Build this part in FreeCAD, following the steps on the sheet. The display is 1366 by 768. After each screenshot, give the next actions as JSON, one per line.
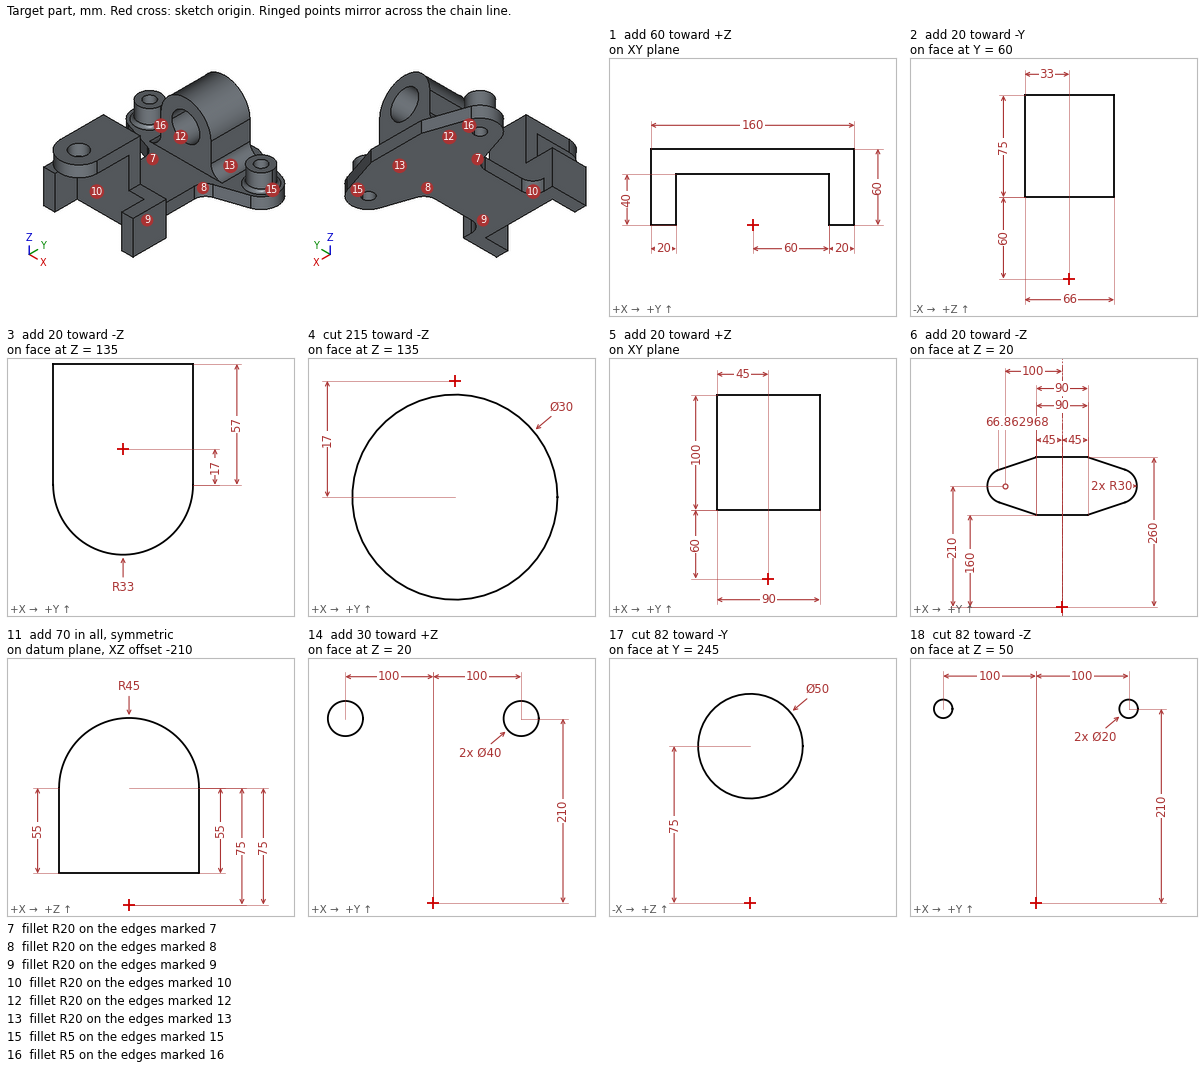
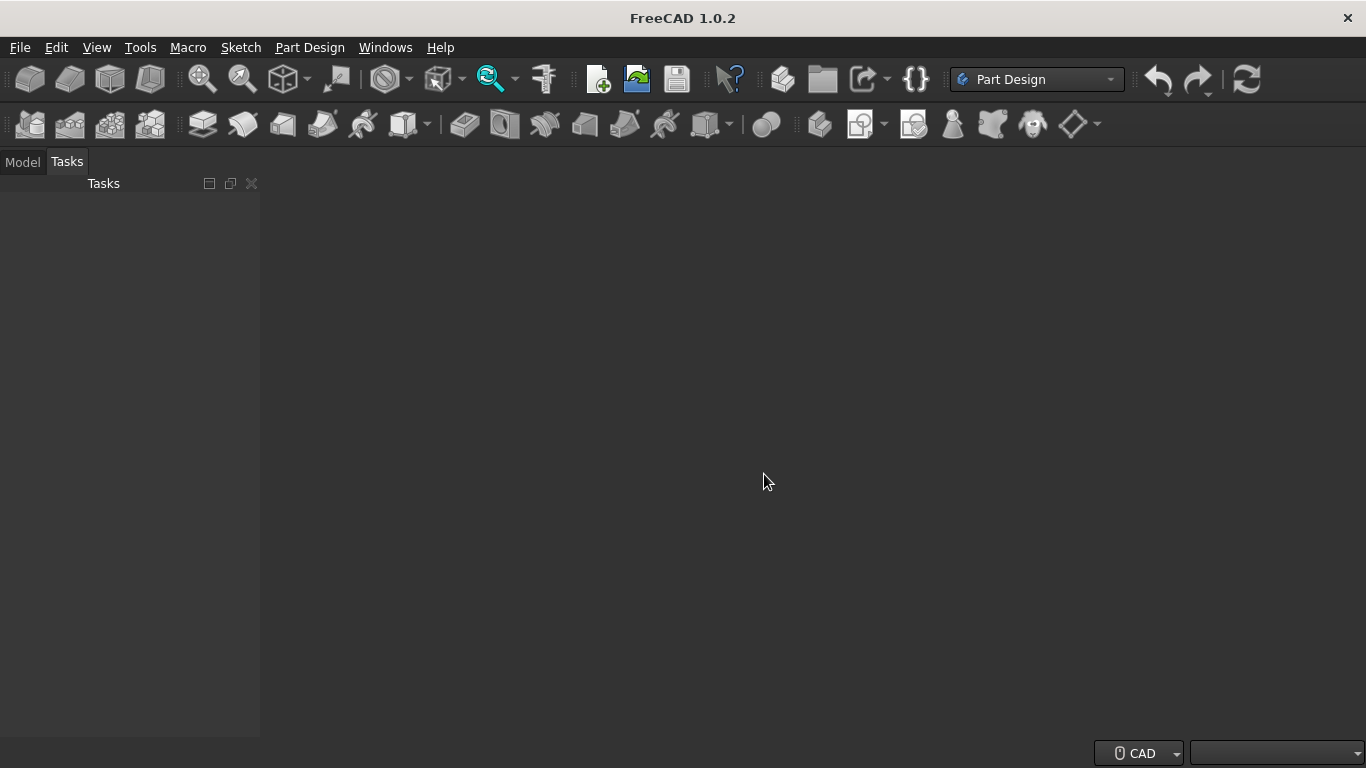
{"action": "key", "text": "ctrl+n"}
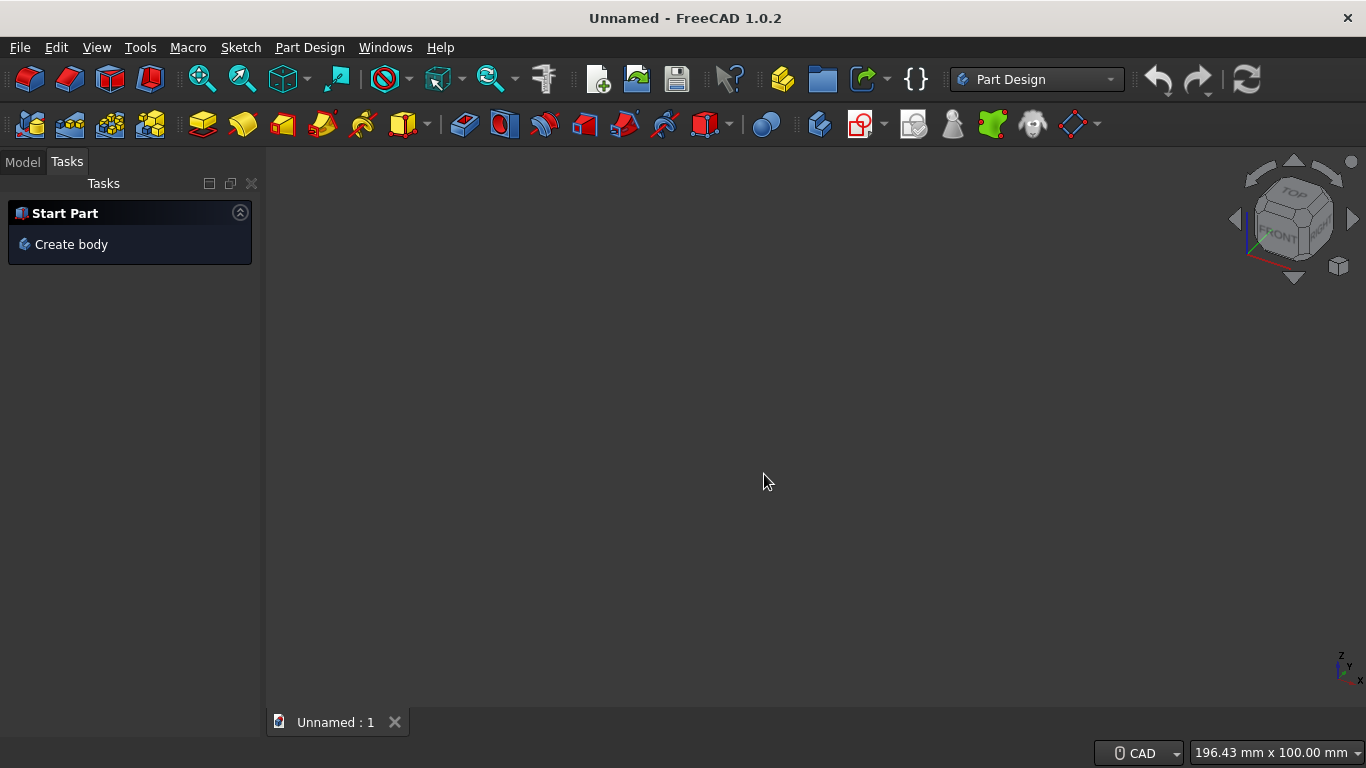
{"action": "left_click", "coordinate": [860, 124]}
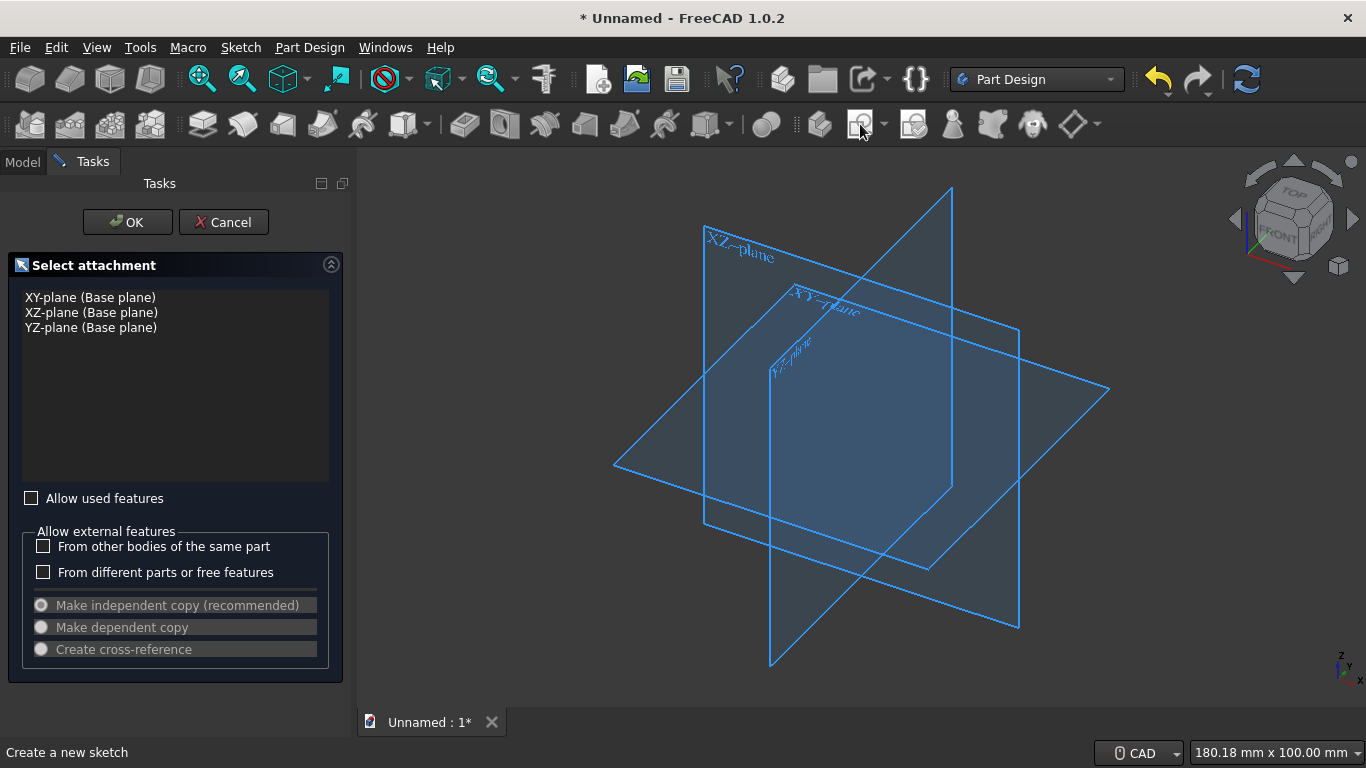
{"action": "left_click", "coordinate": [82, 298]}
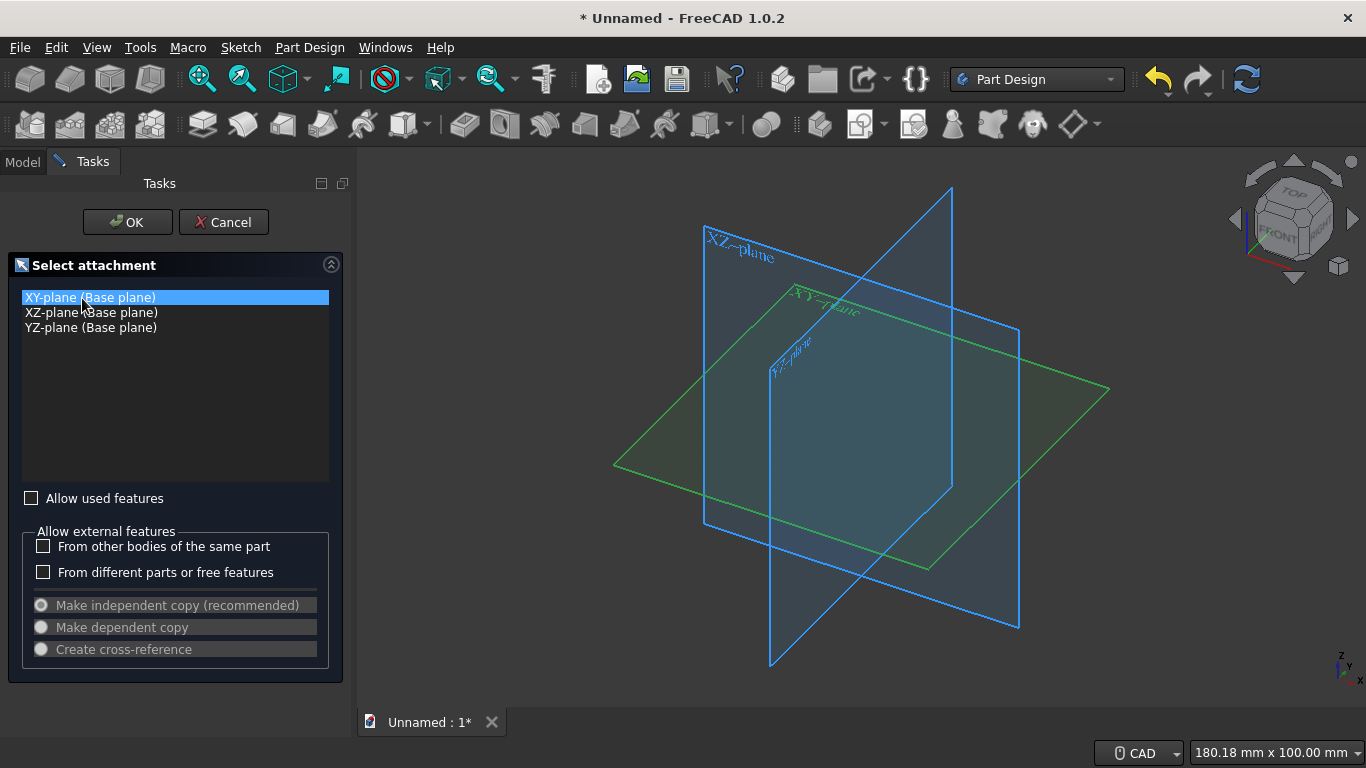
{"action": "left_click", "coordinate": [128, 222]}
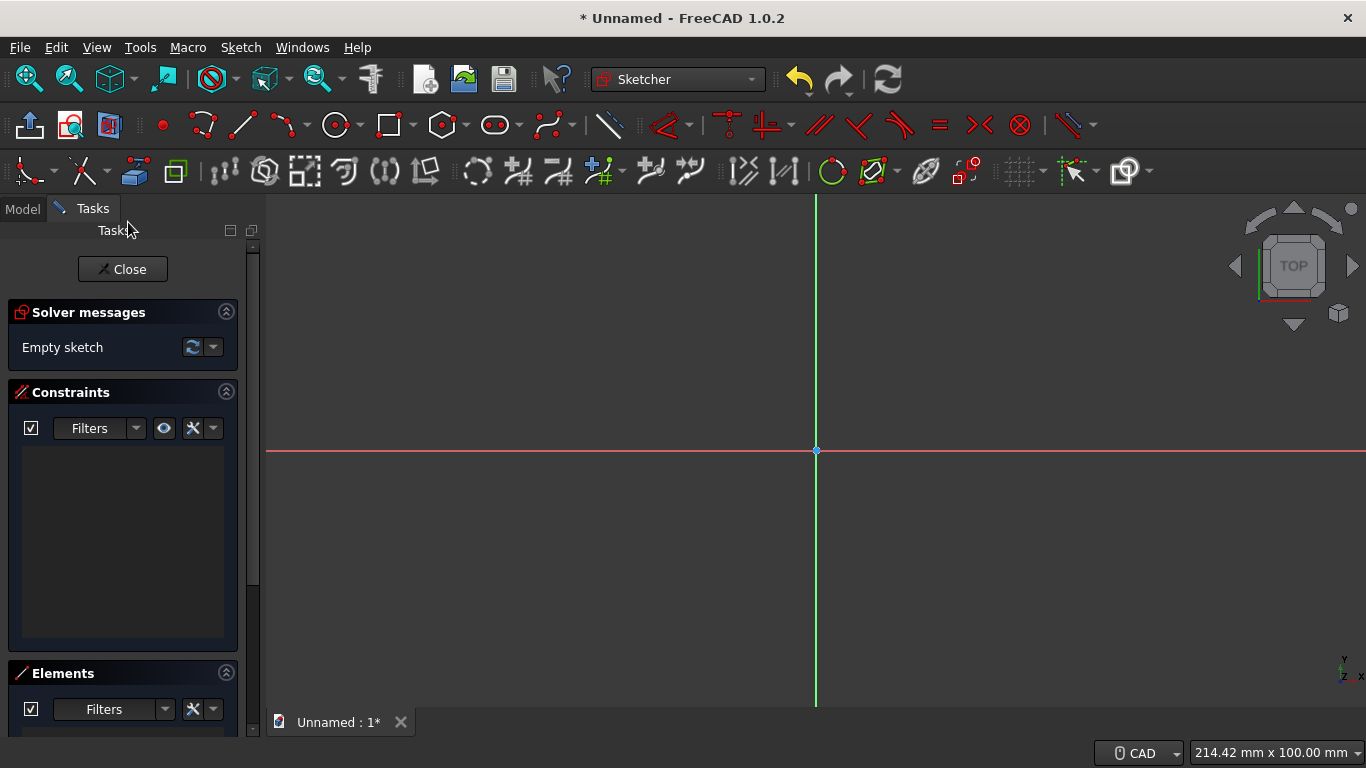
{"action": "scroll", "coordinate": [608, 679], "scroll_direction": "down", "scroll_amount": 2}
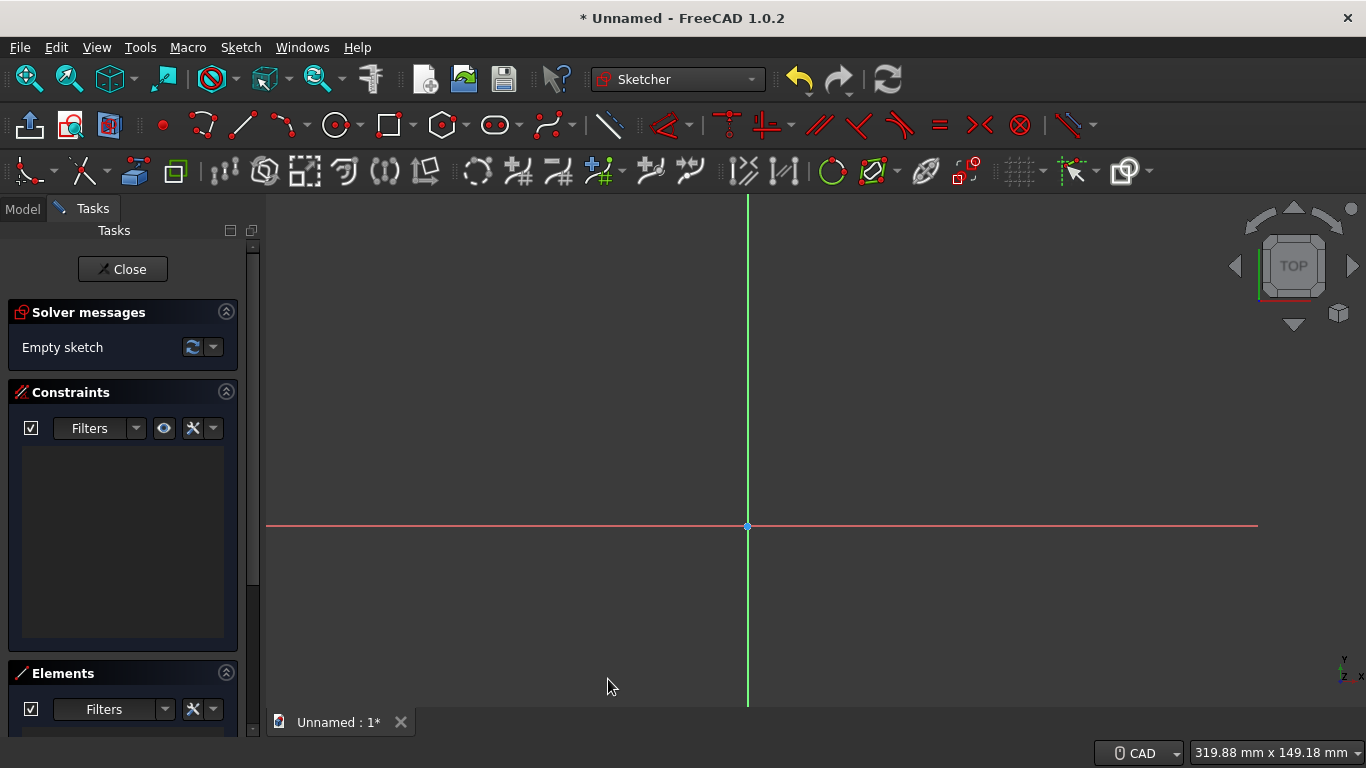
{"action": "key", "text": "g m"}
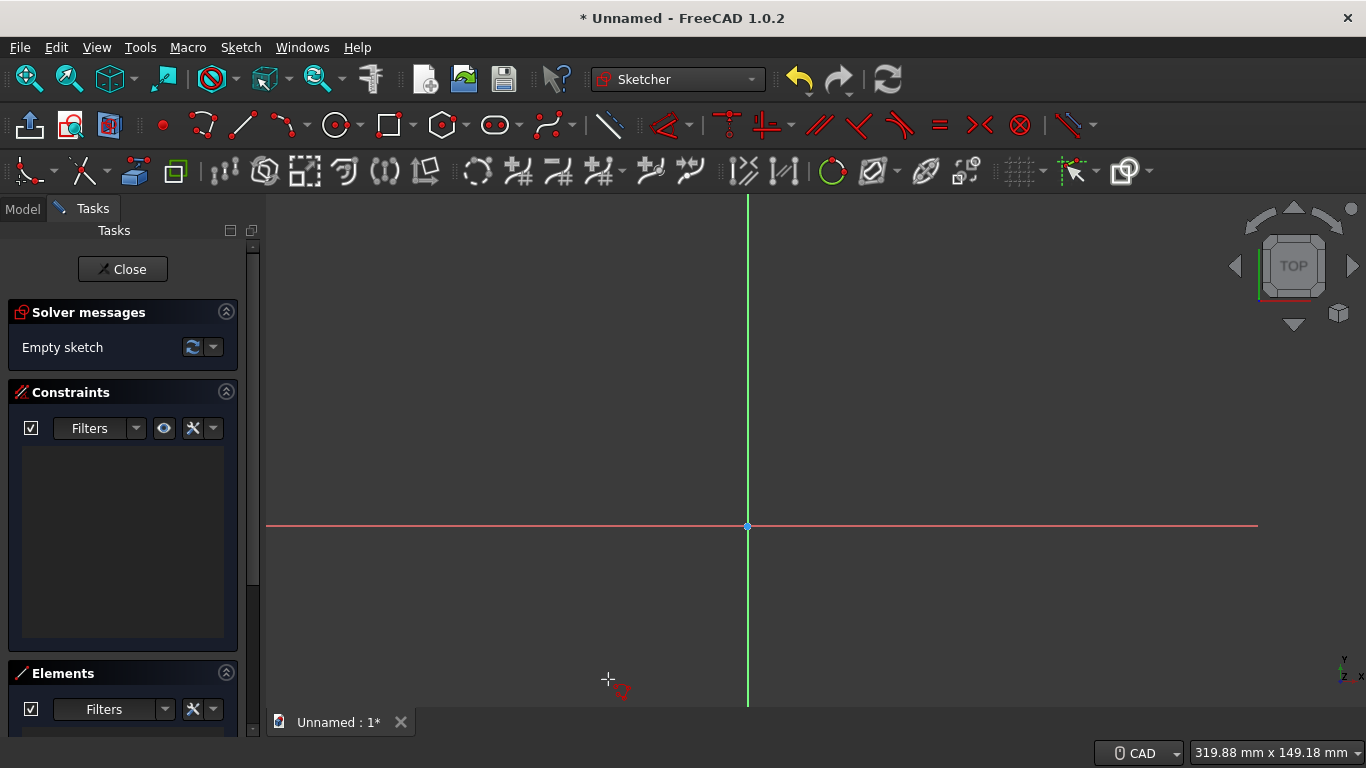
{"action": "left_click", "coordinate": [954, 526]}
{"action": "left_click", "coordinate": [1023, 517]}
{"action": "left_click", "coordinate": [1023, 320]}
{"action": "left_click", "coordinate": [472, 320]}
{"action": "left_click", "coordinate": [472, 526]}
{"action": "left_click", "coordinate": [541, 517]}
{"action": "left_click", "coordinate": [541, 389]}
{"action": "left_click", "coordinate": [954, 389]}
{"action": "left_click", "coordinate": [954, 526]}
{"action": "key", "text": "Escape"}
{"action": "key", "text": "Escape"}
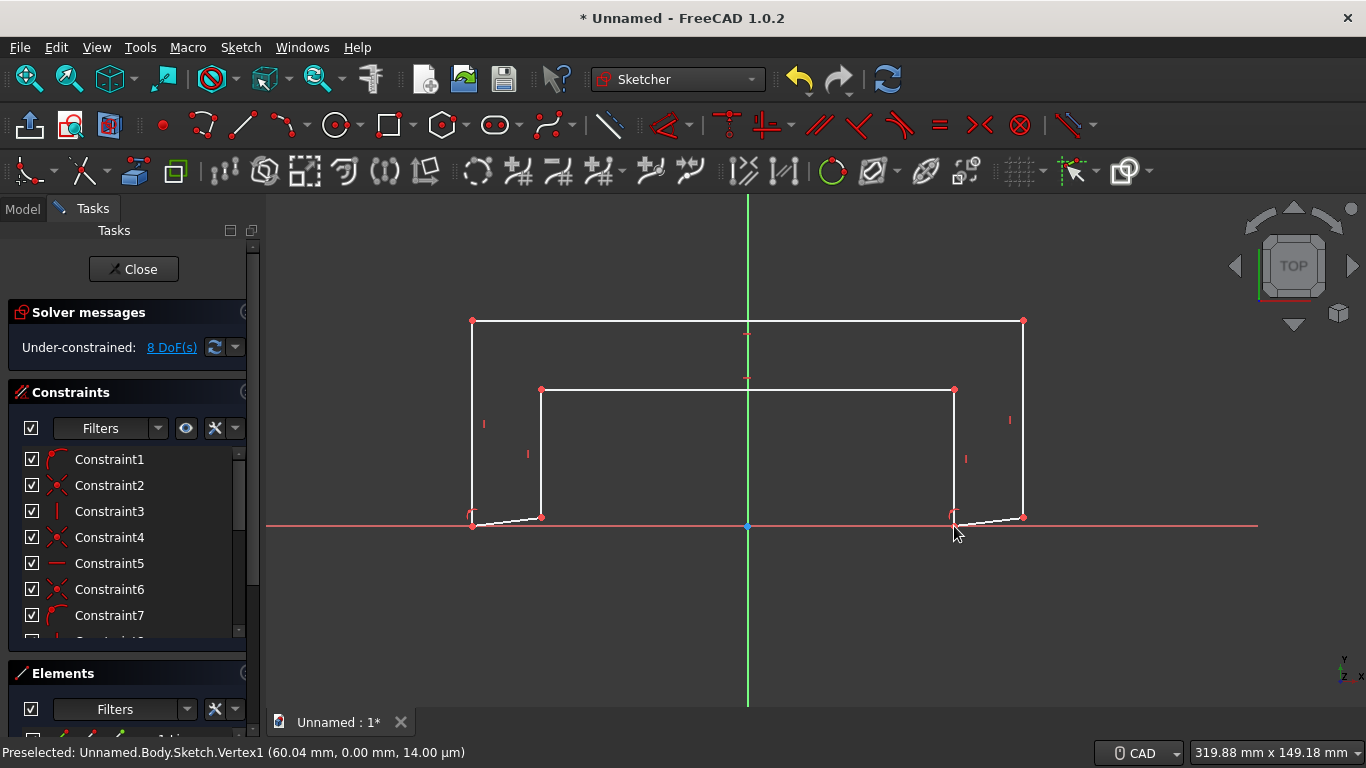
{"action": "left_click", "coordinate": [975, 524]}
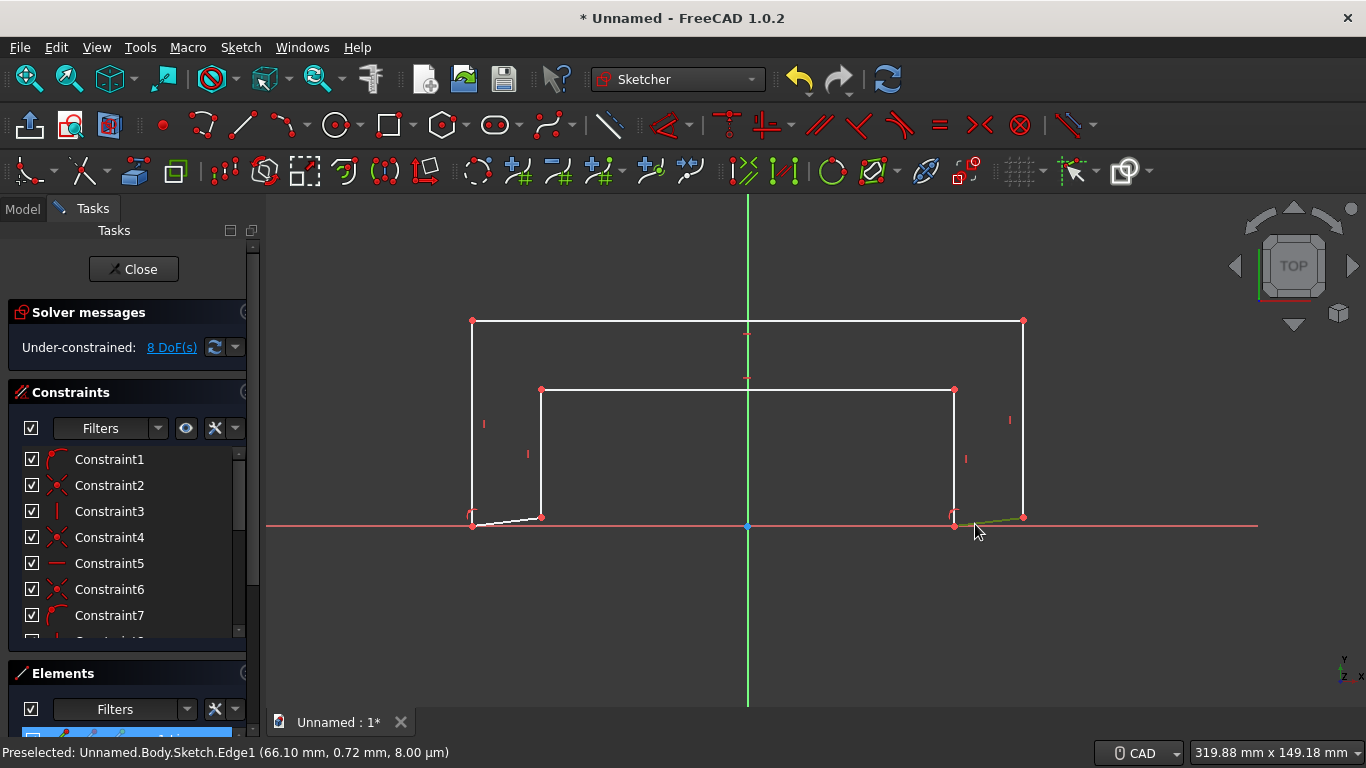
{"action": "key", "text": "h"}